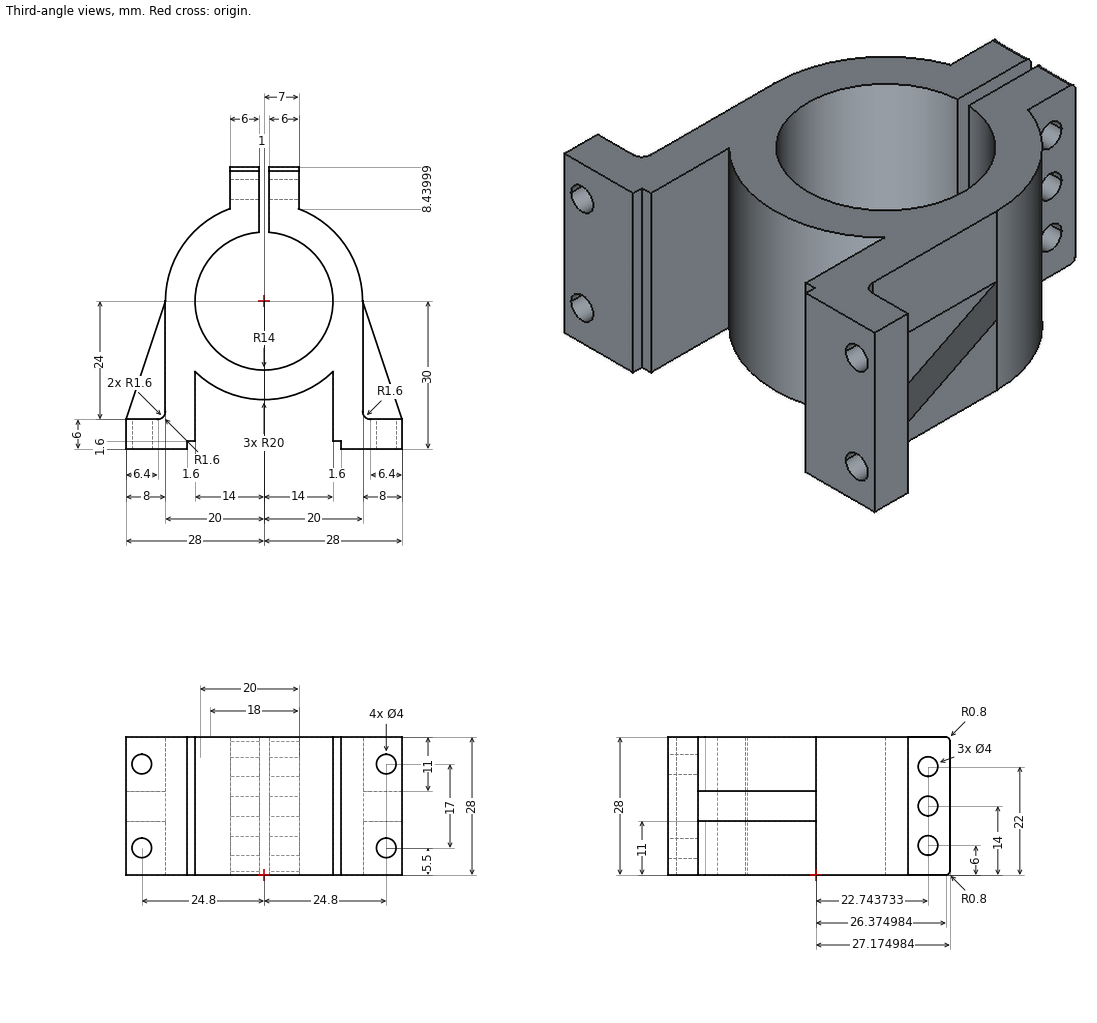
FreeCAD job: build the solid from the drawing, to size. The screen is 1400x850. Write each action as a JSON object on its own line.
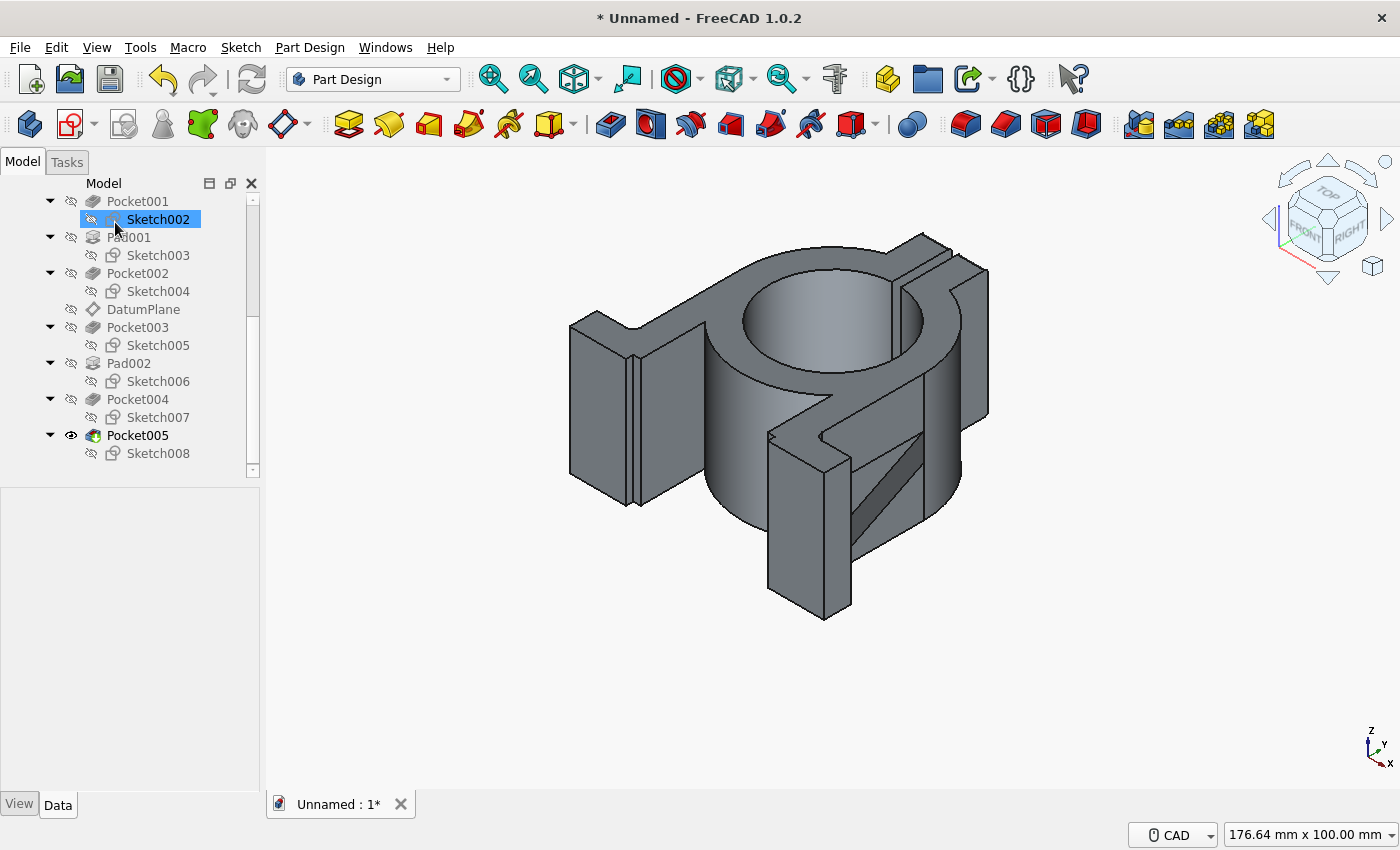
{"action": "left_click", "coordinate": [969, 310]}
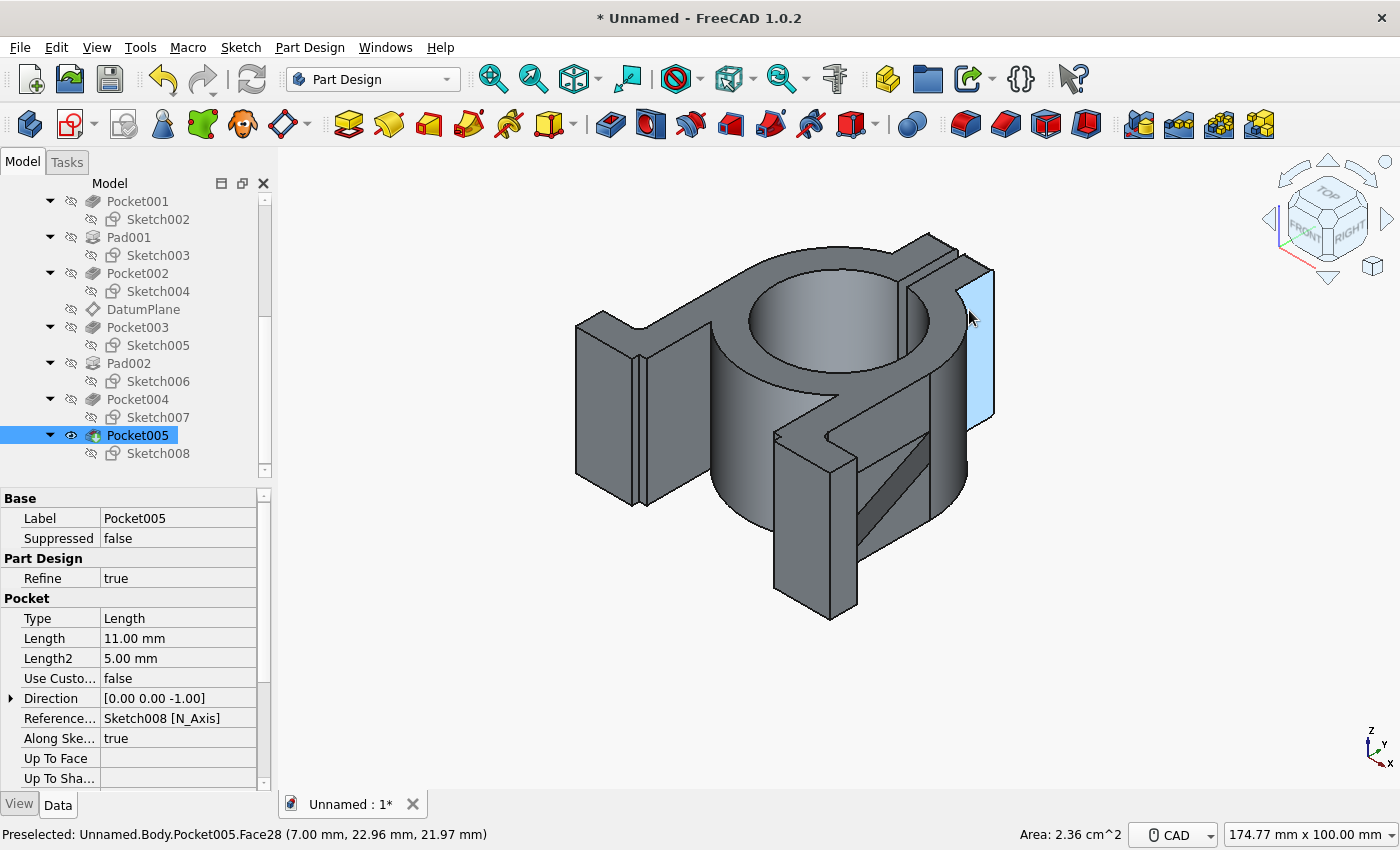
{"action": "left_click", "coordinate": [70, 124]}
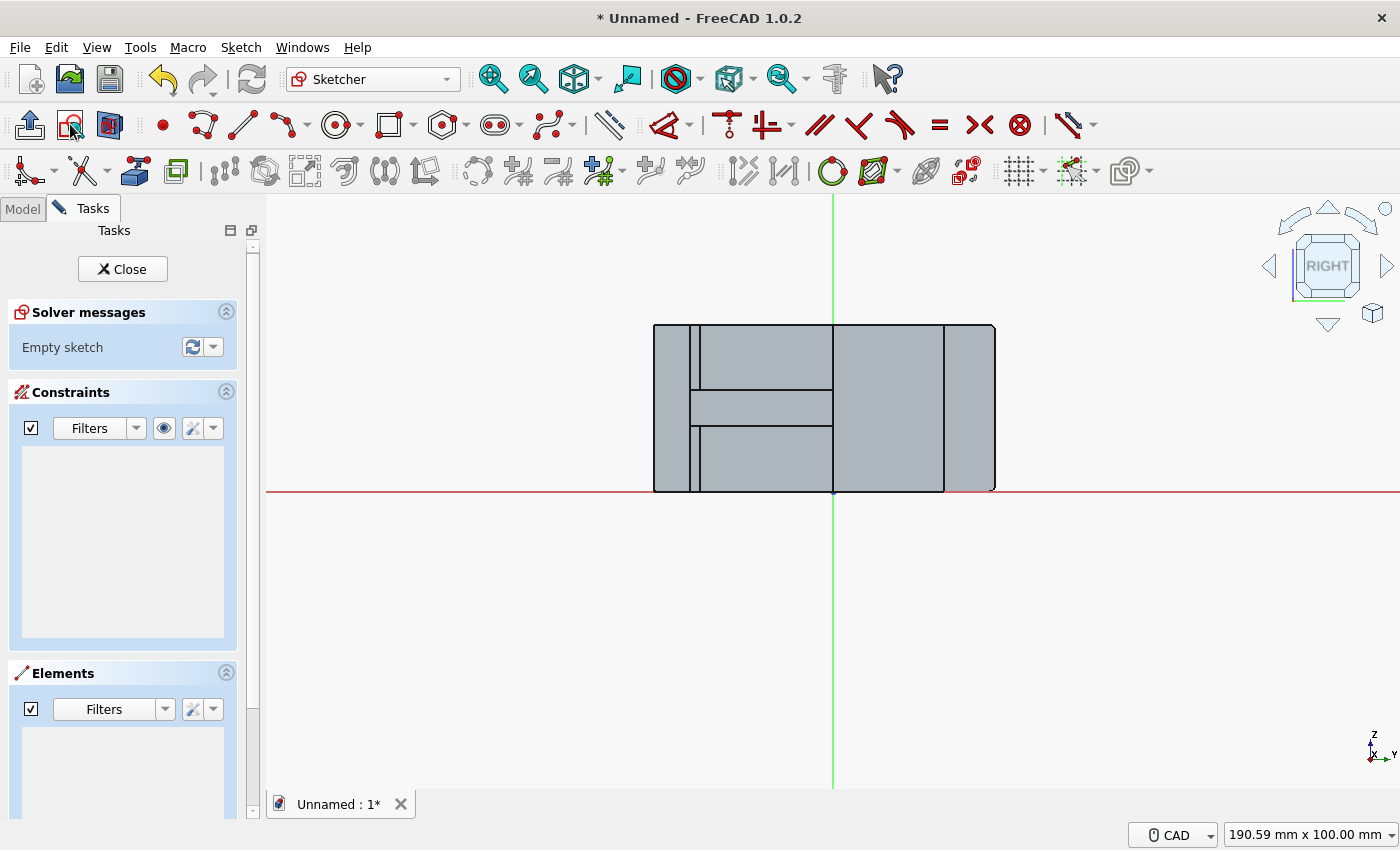
{"action": "left_click", "coordinate": [110, 126]}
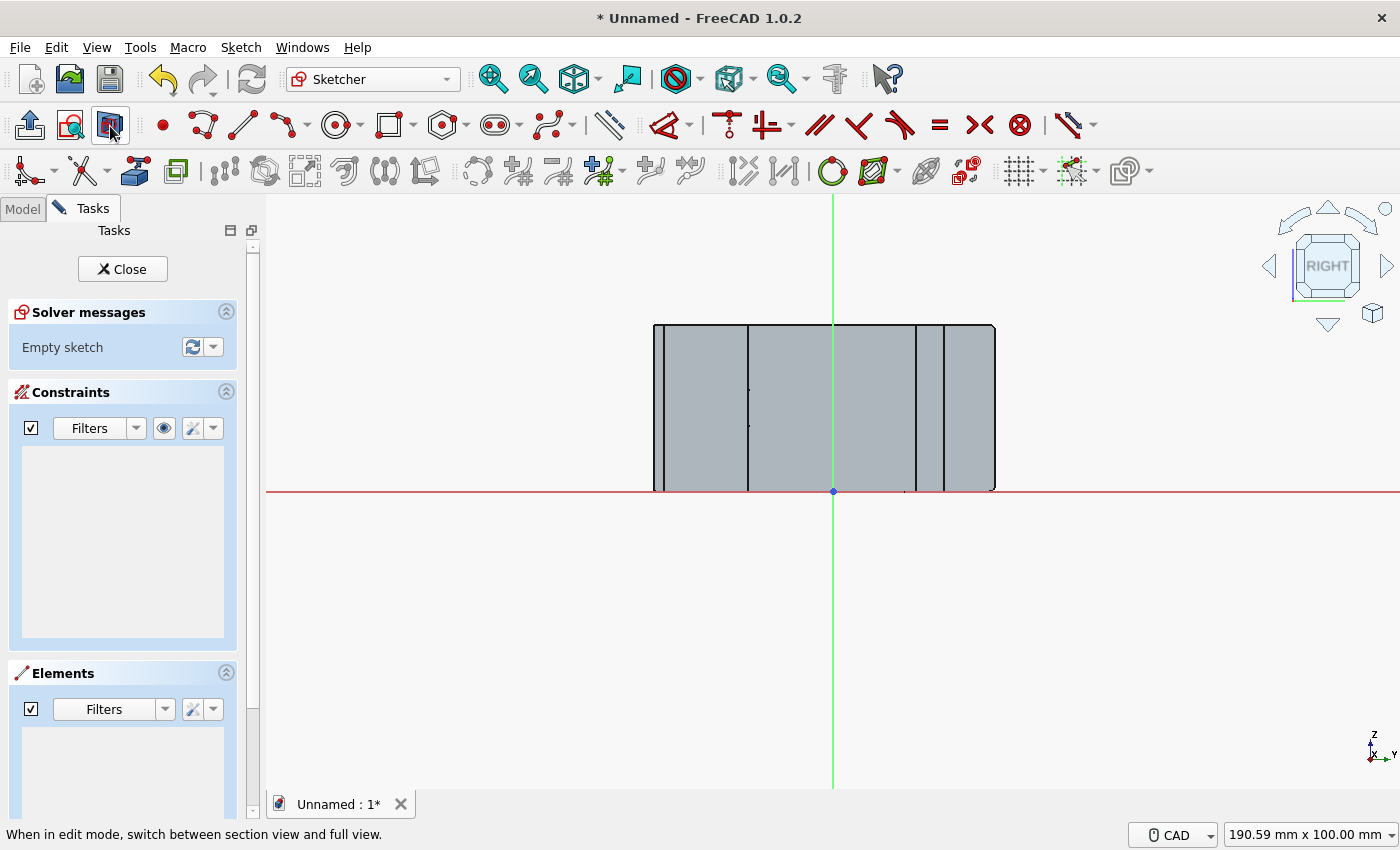
{"action": "scroll", "coordinate": [989, 379], "scroll_direction": "up", "scroll_amount": 5}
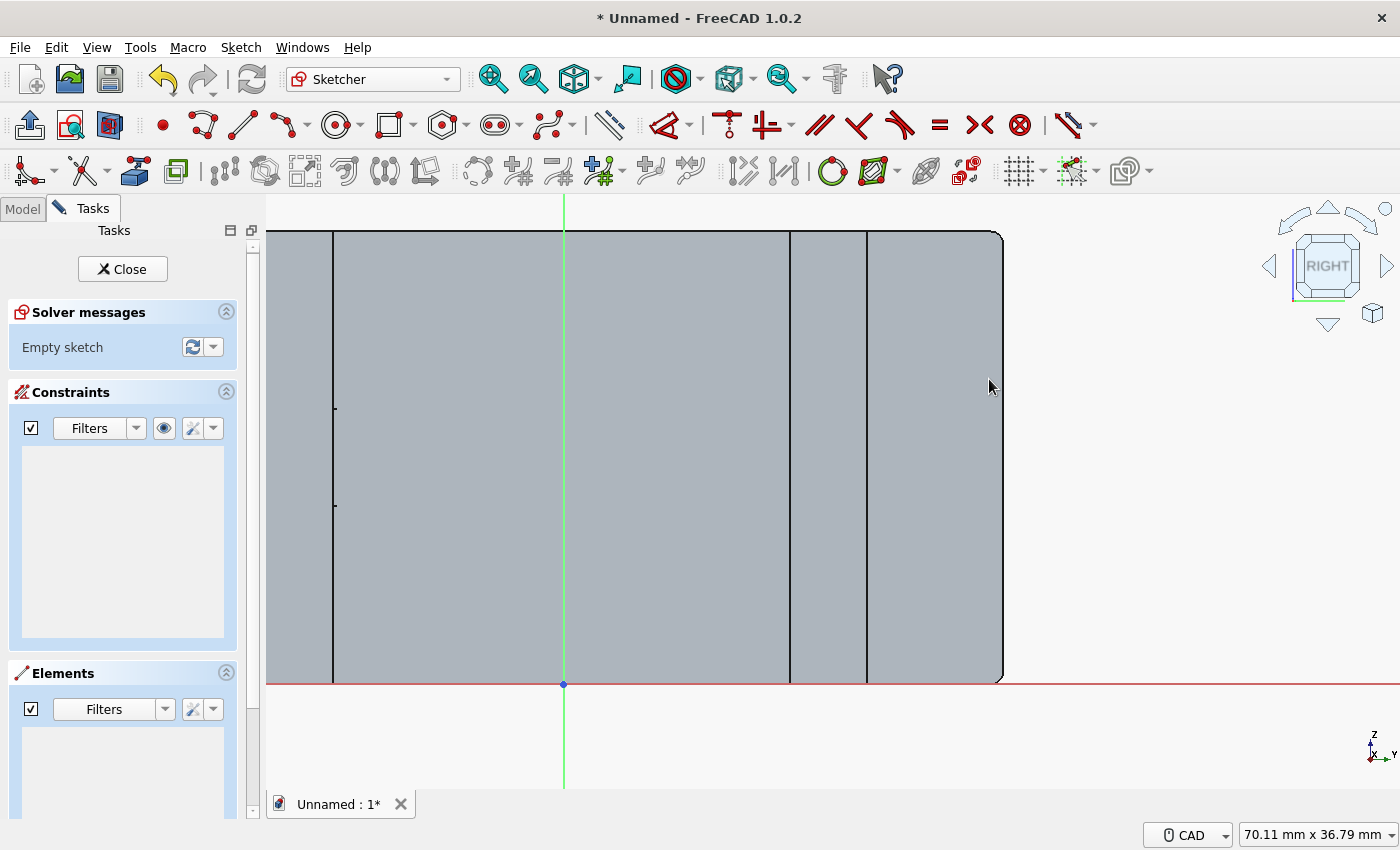
{"action": "left_click", "coordinate": [336, 126]}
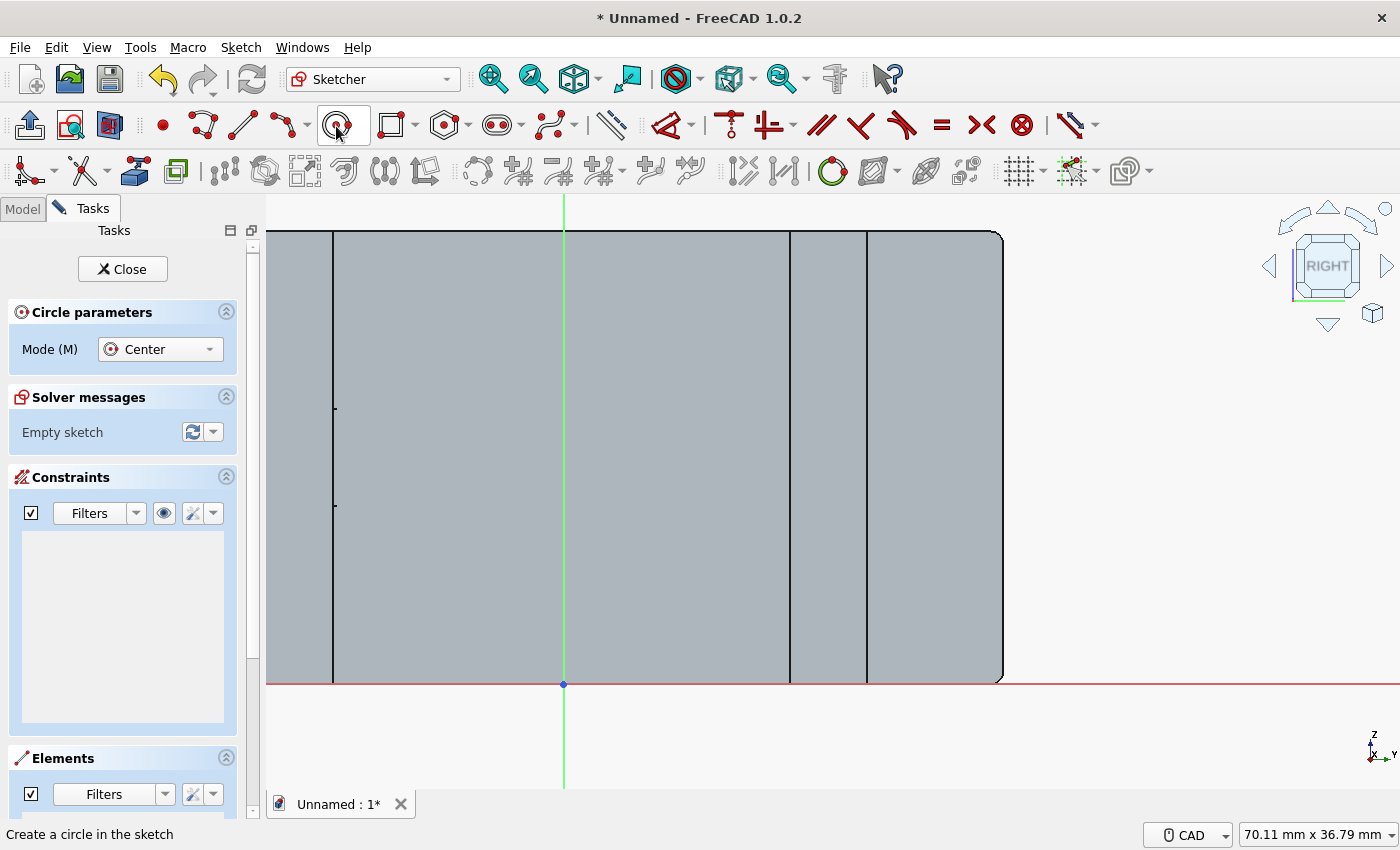
{"action": "left_click", "coordinate": [932, 328]}
{"action": "mouse_move", "coordinate": [955, 306]}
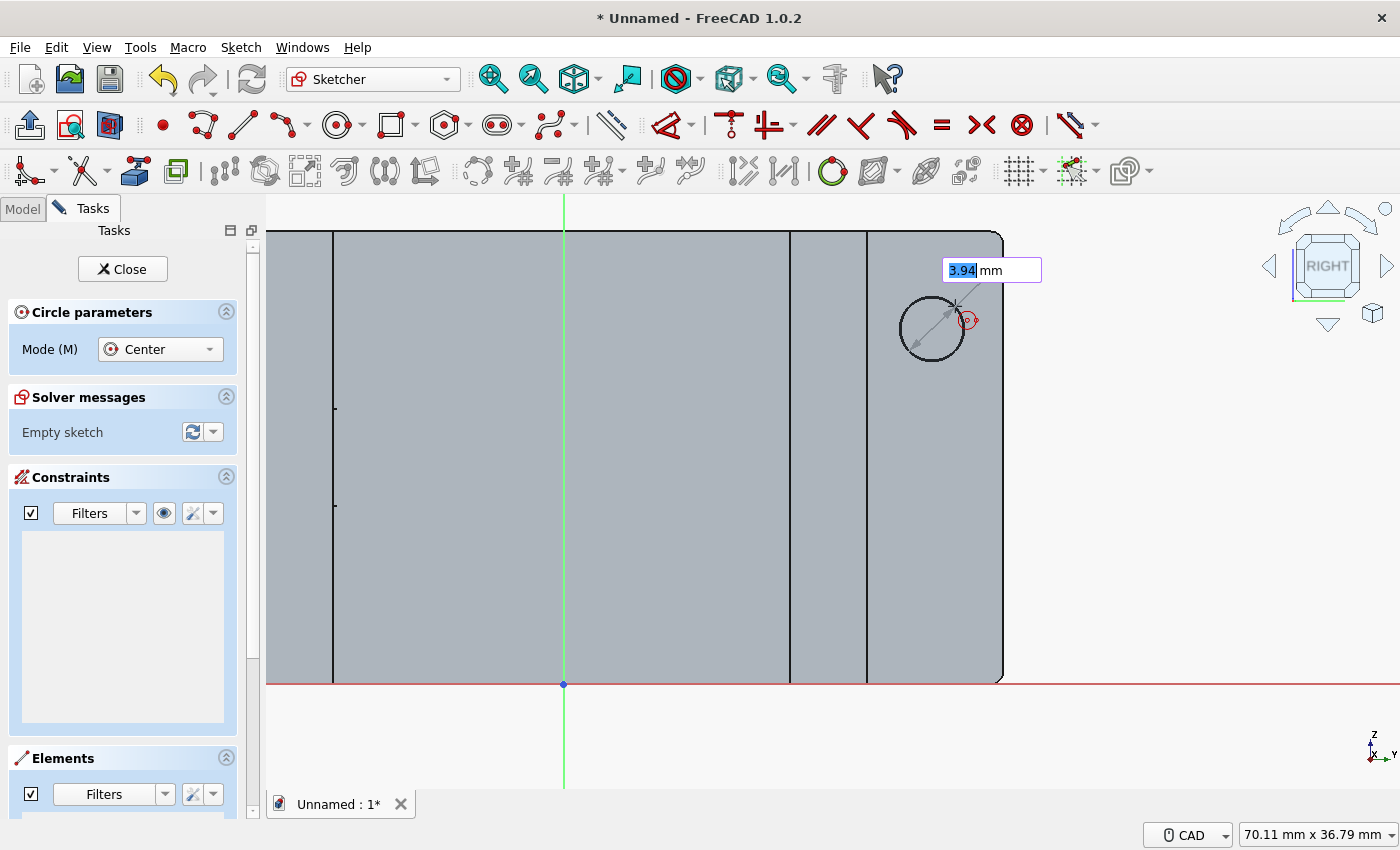
{"action": "type", "text": "4"}
{"action": "key", "text": "Return"}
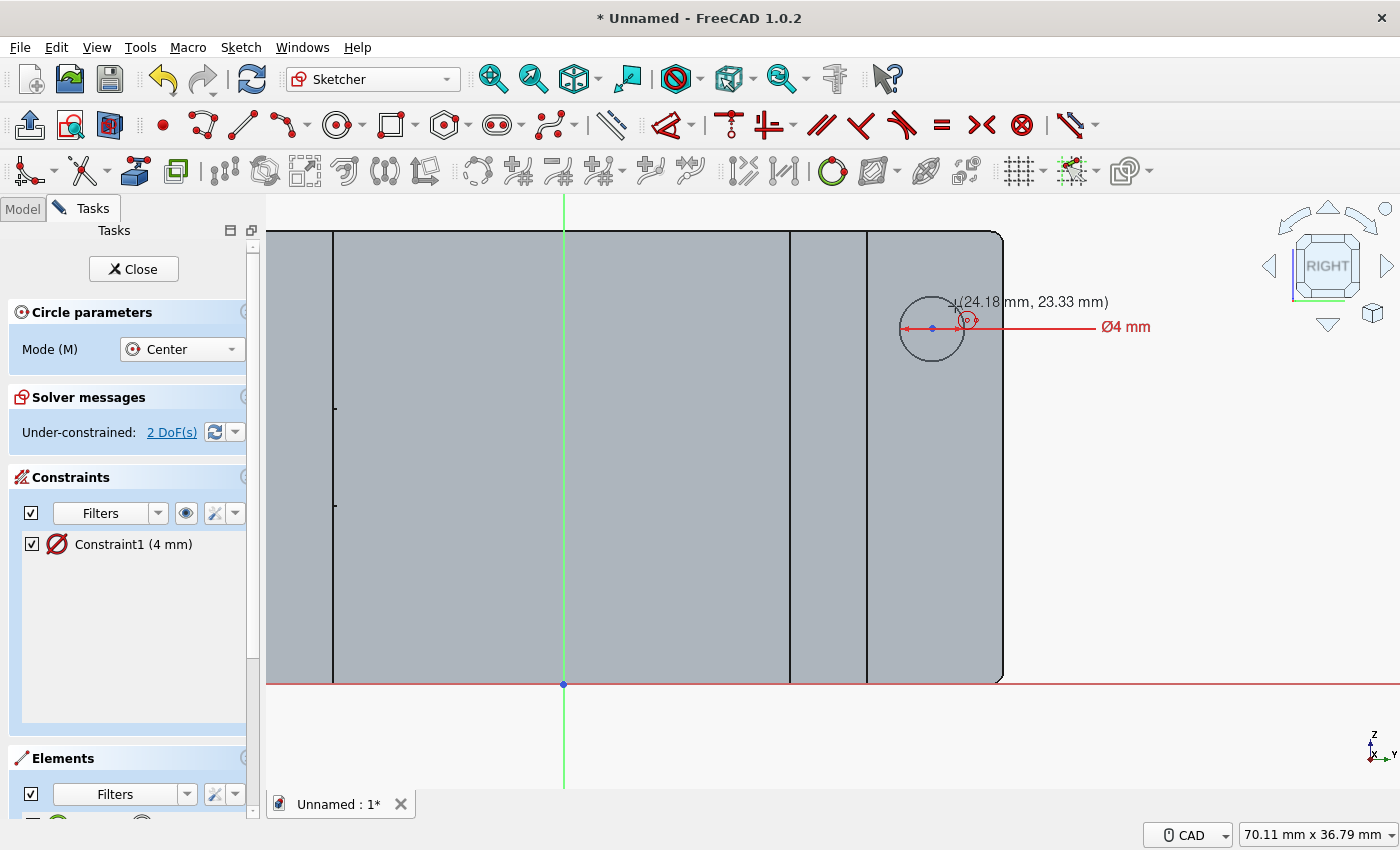
{"action": "left_click", "coordinate": [932, 458]}
{"action": "mouse_move", "coordinate": [955, 435]}